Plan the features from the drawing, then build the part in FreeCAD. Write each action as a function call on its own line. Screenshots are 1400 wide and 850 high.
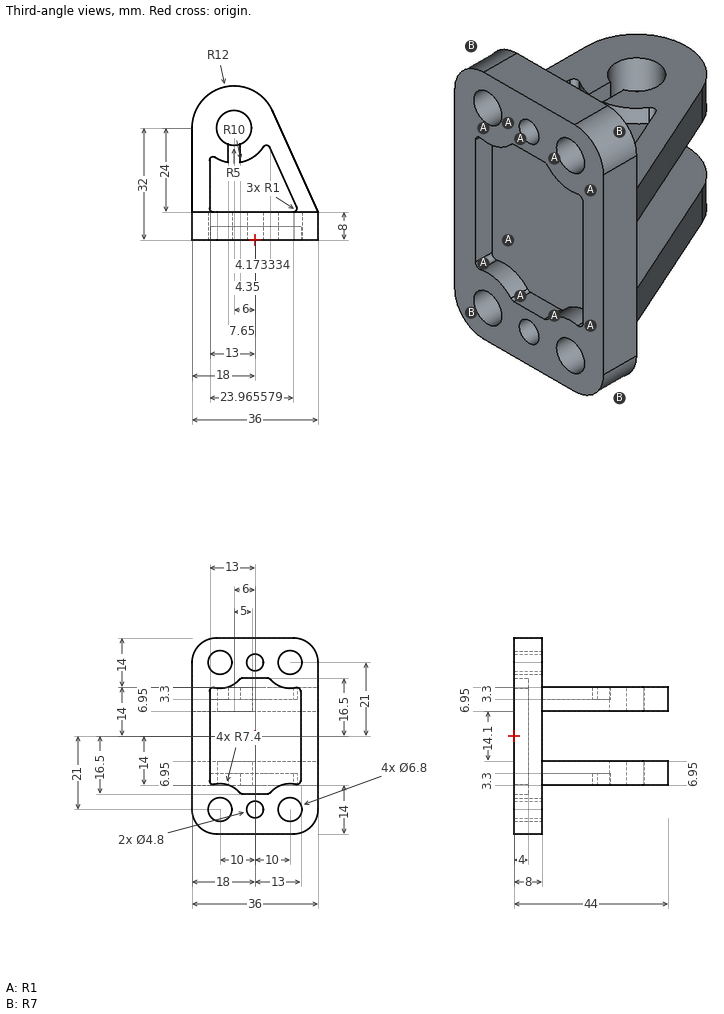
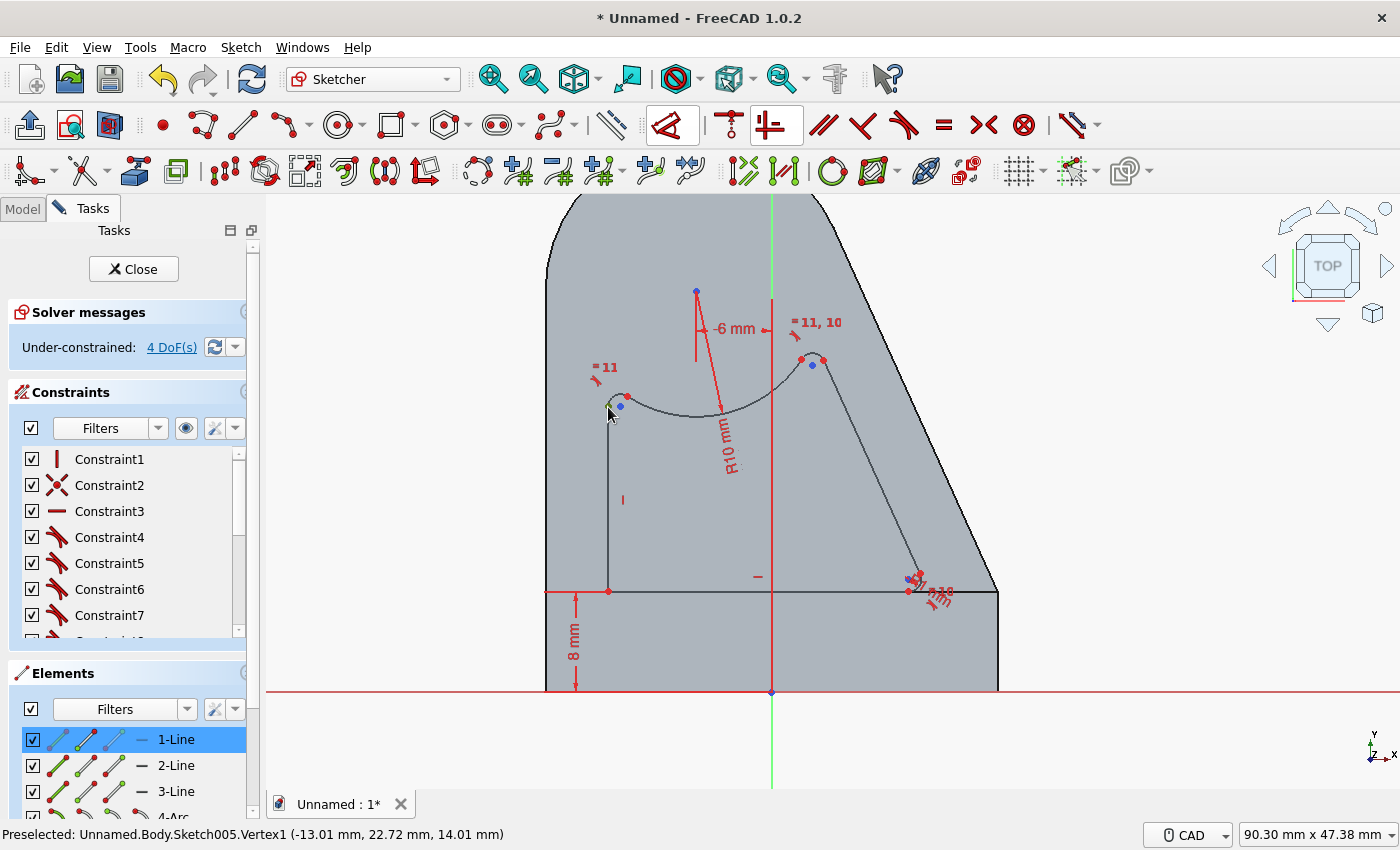
key(l)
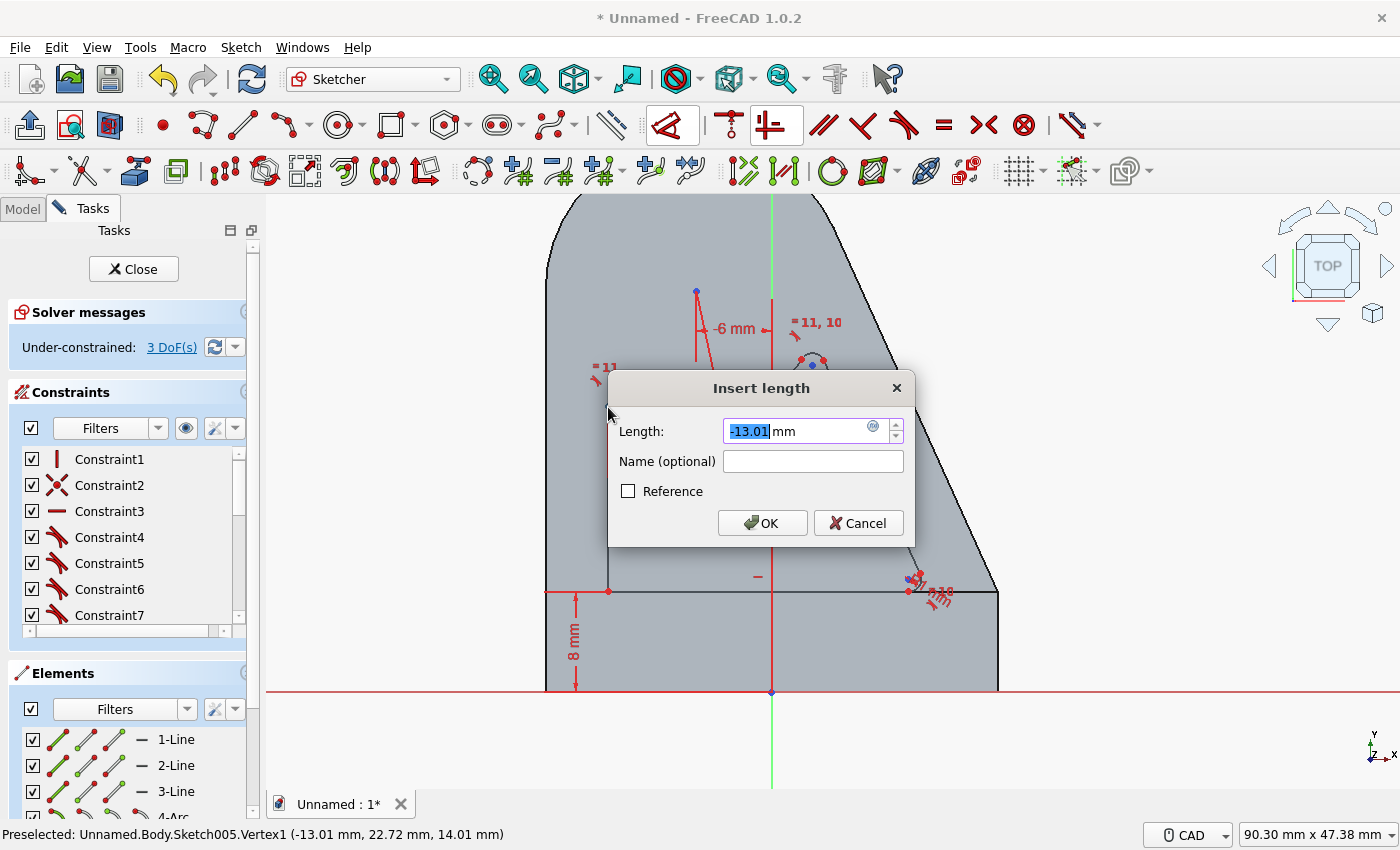
text(-13)
key(Return)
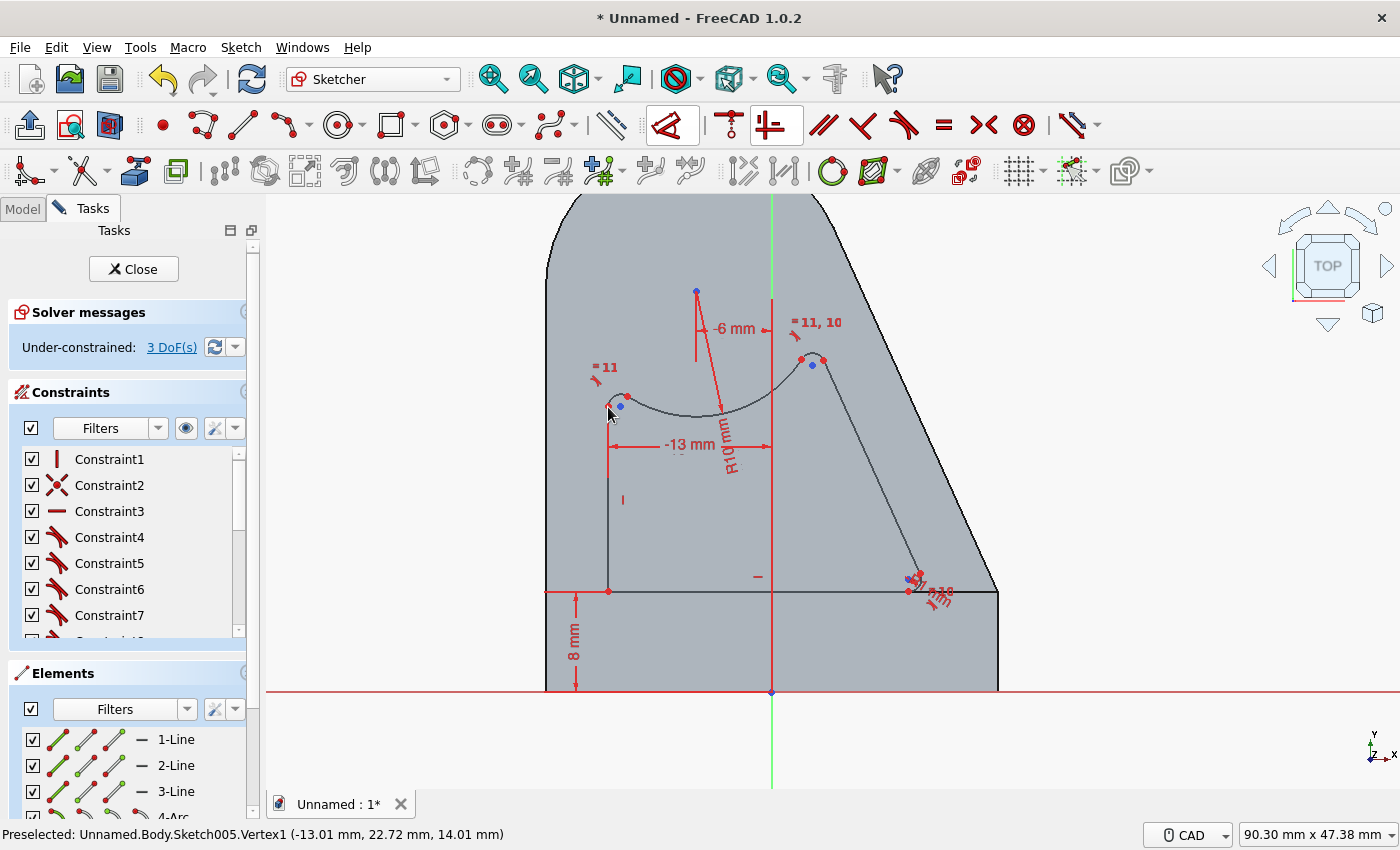
click(696, 291)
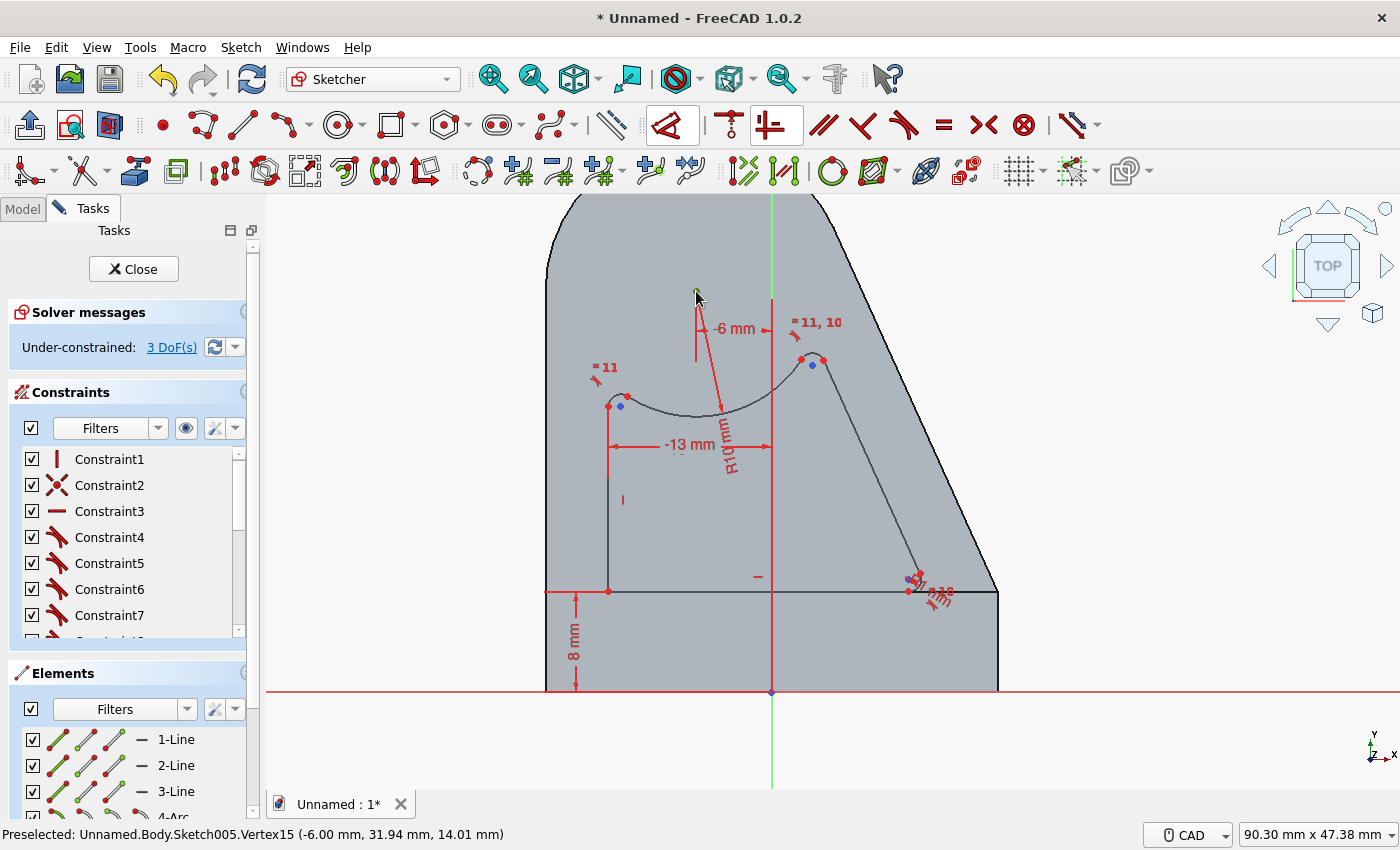
key(i)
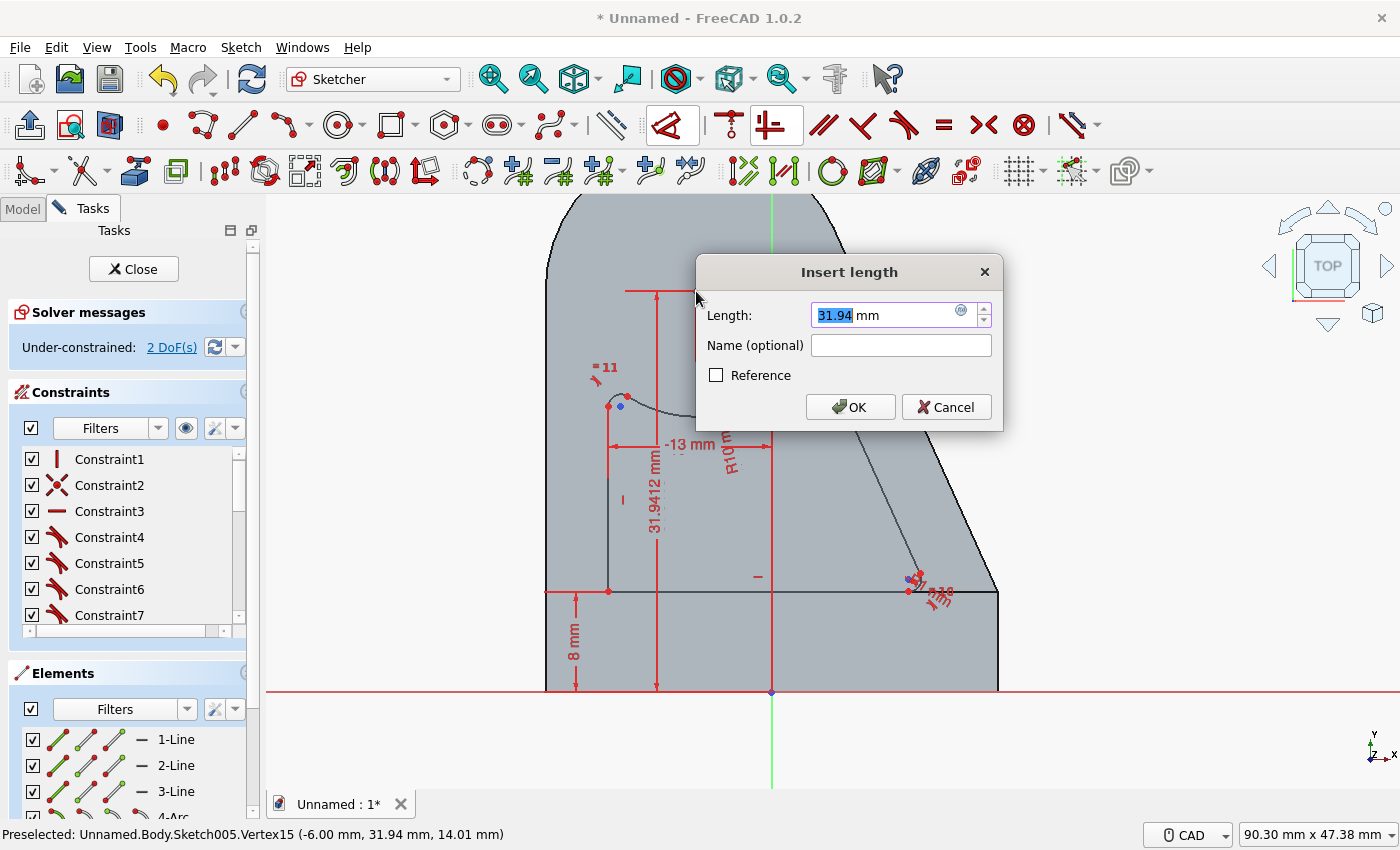
text(32)
key(Return)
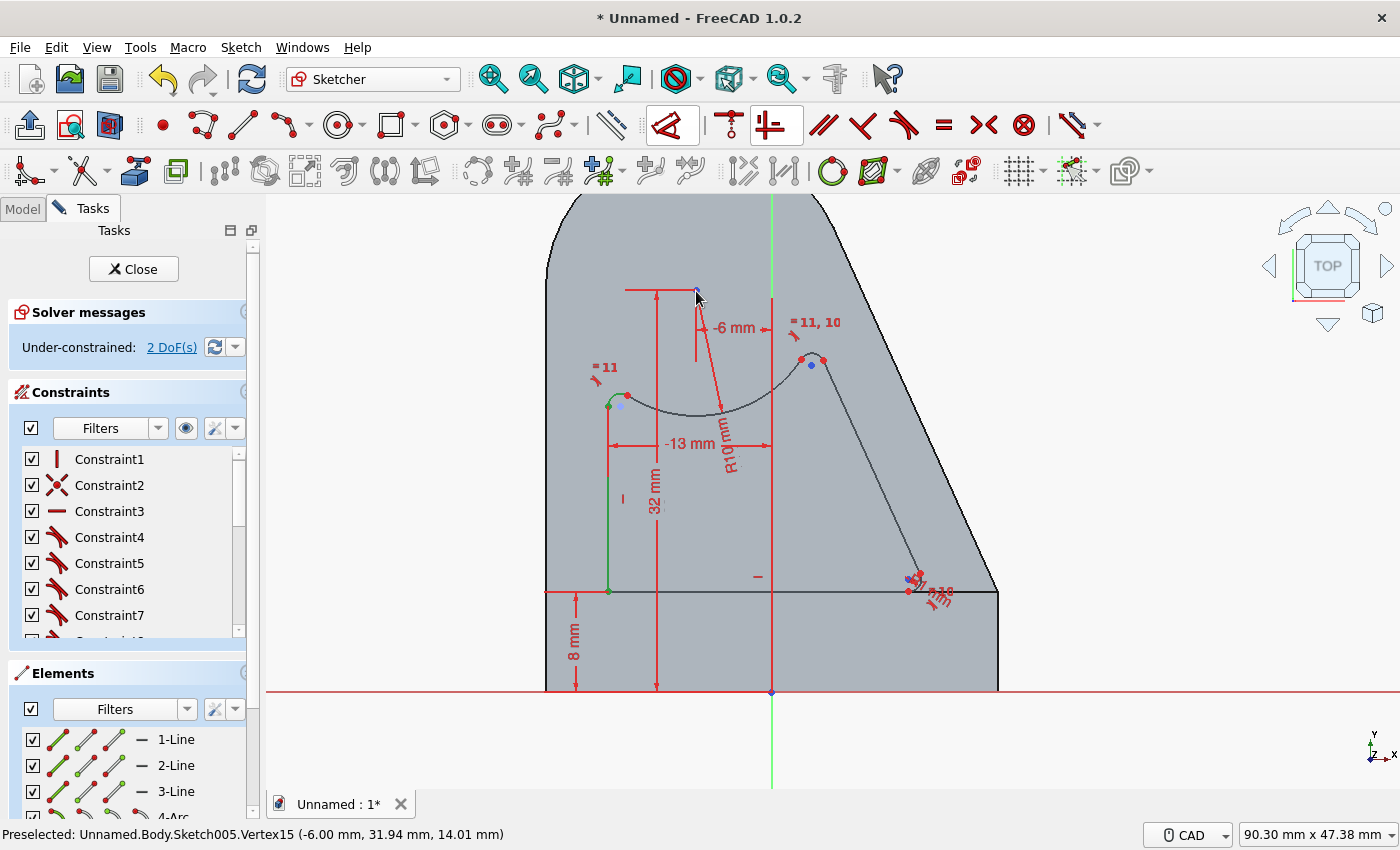
click(699, 592)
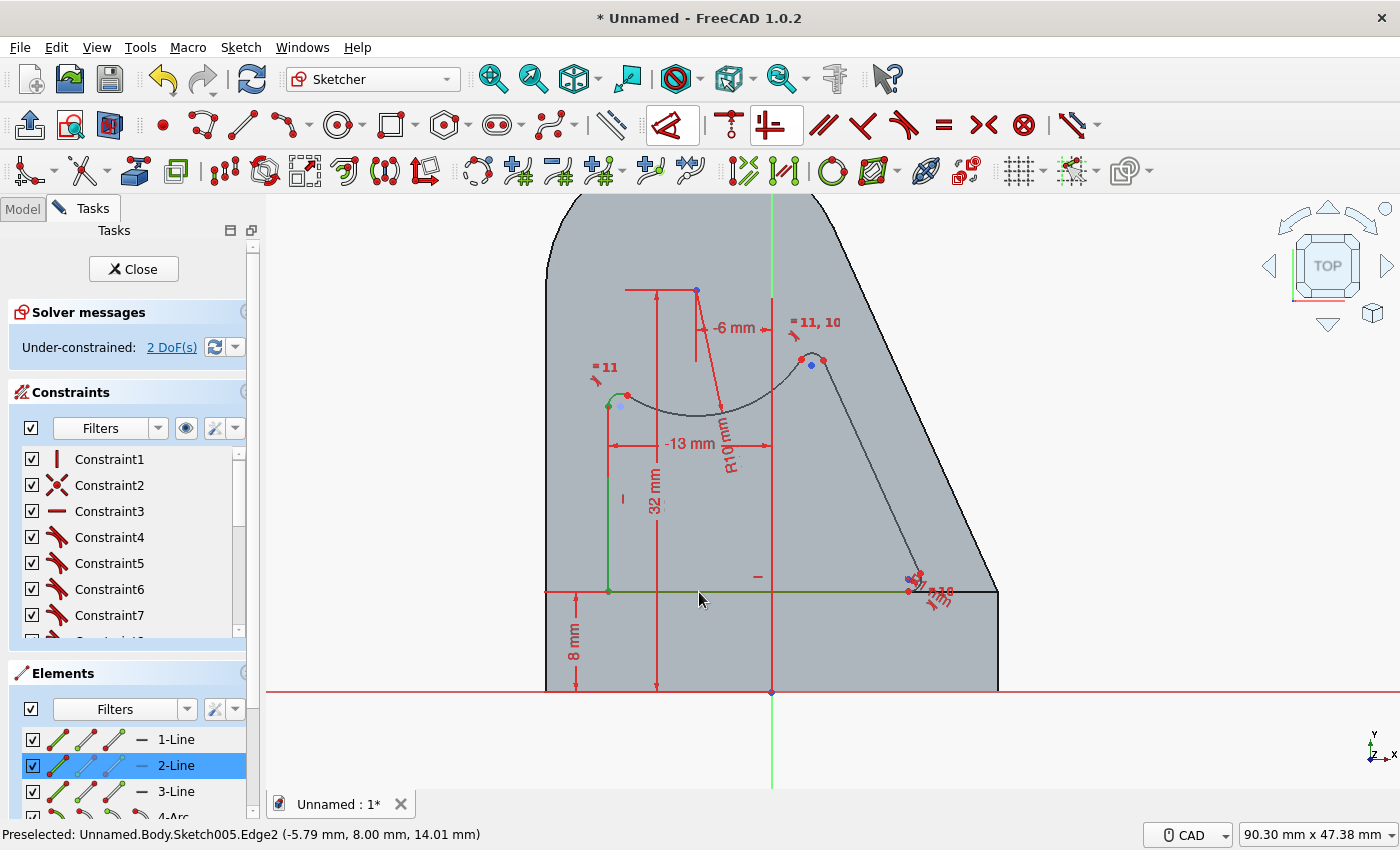
key(l)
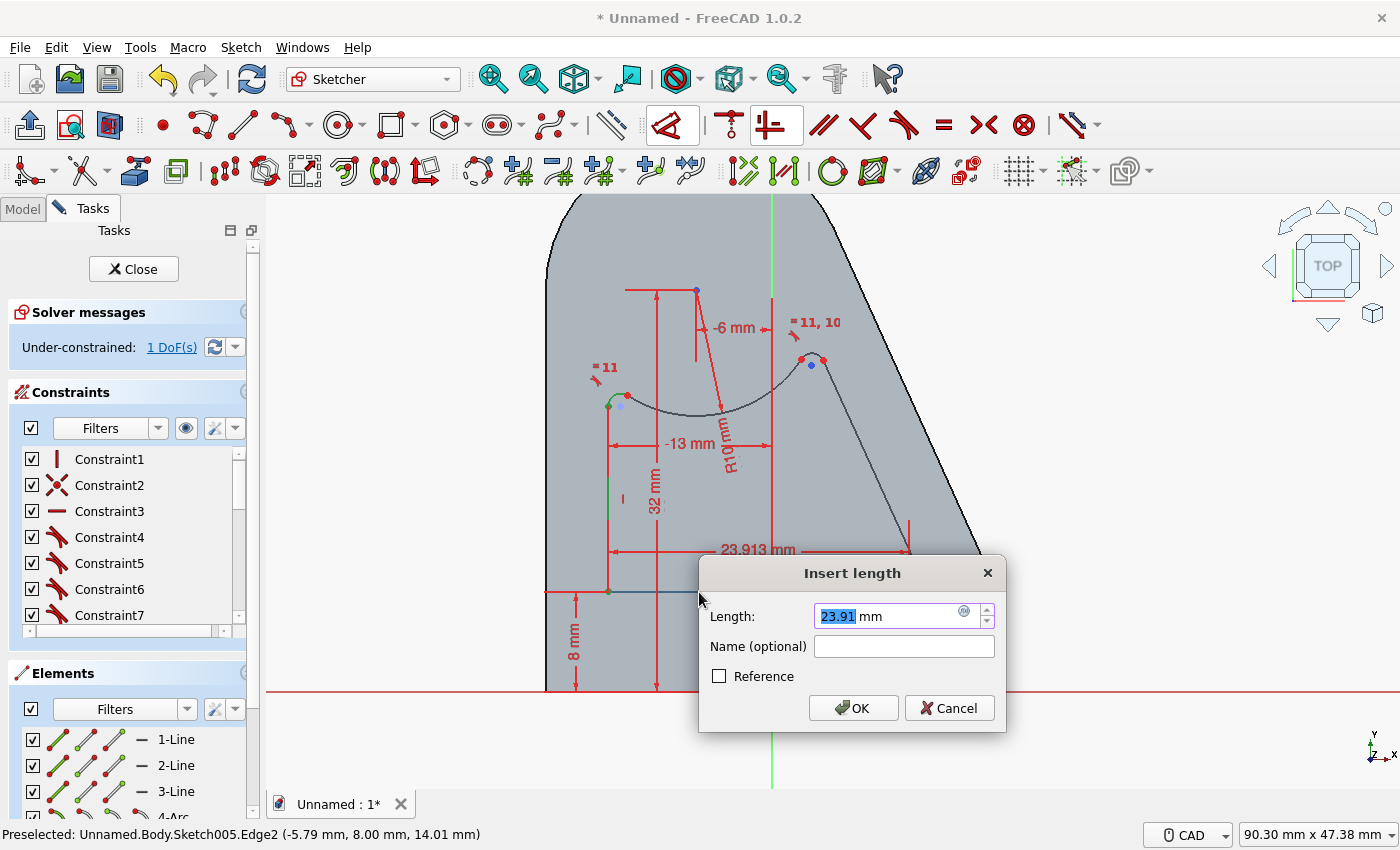
text(23.965579)
key(Return)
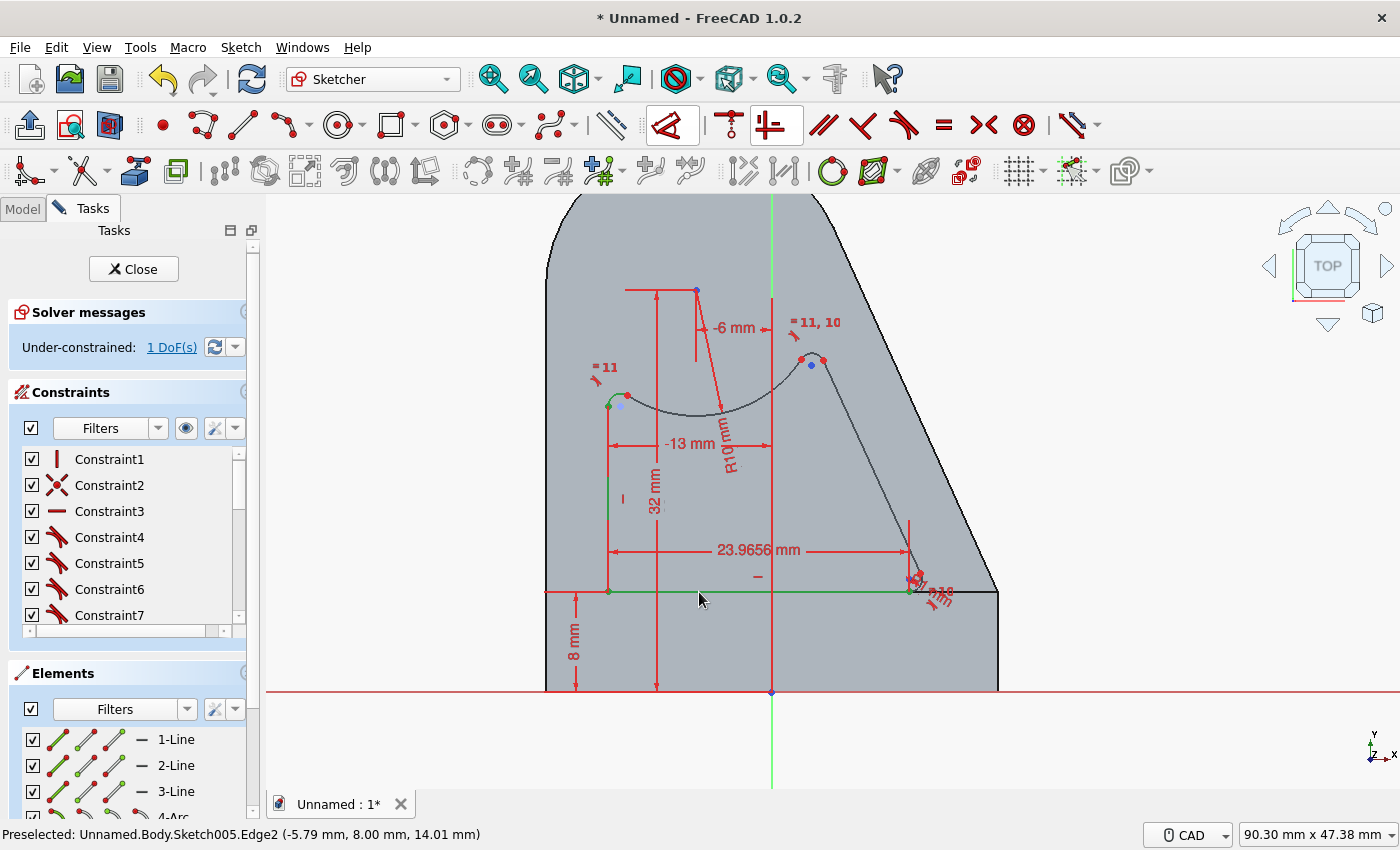
click(823, 361)